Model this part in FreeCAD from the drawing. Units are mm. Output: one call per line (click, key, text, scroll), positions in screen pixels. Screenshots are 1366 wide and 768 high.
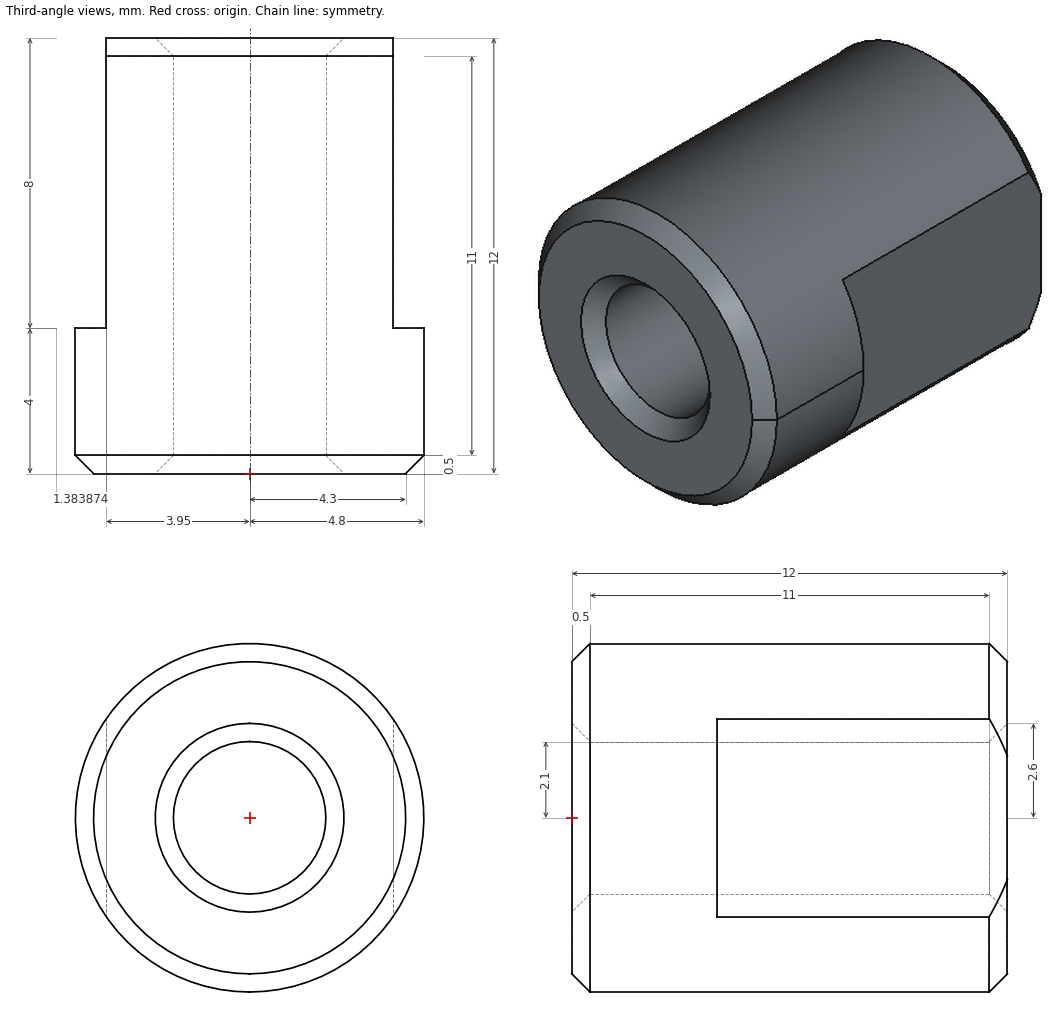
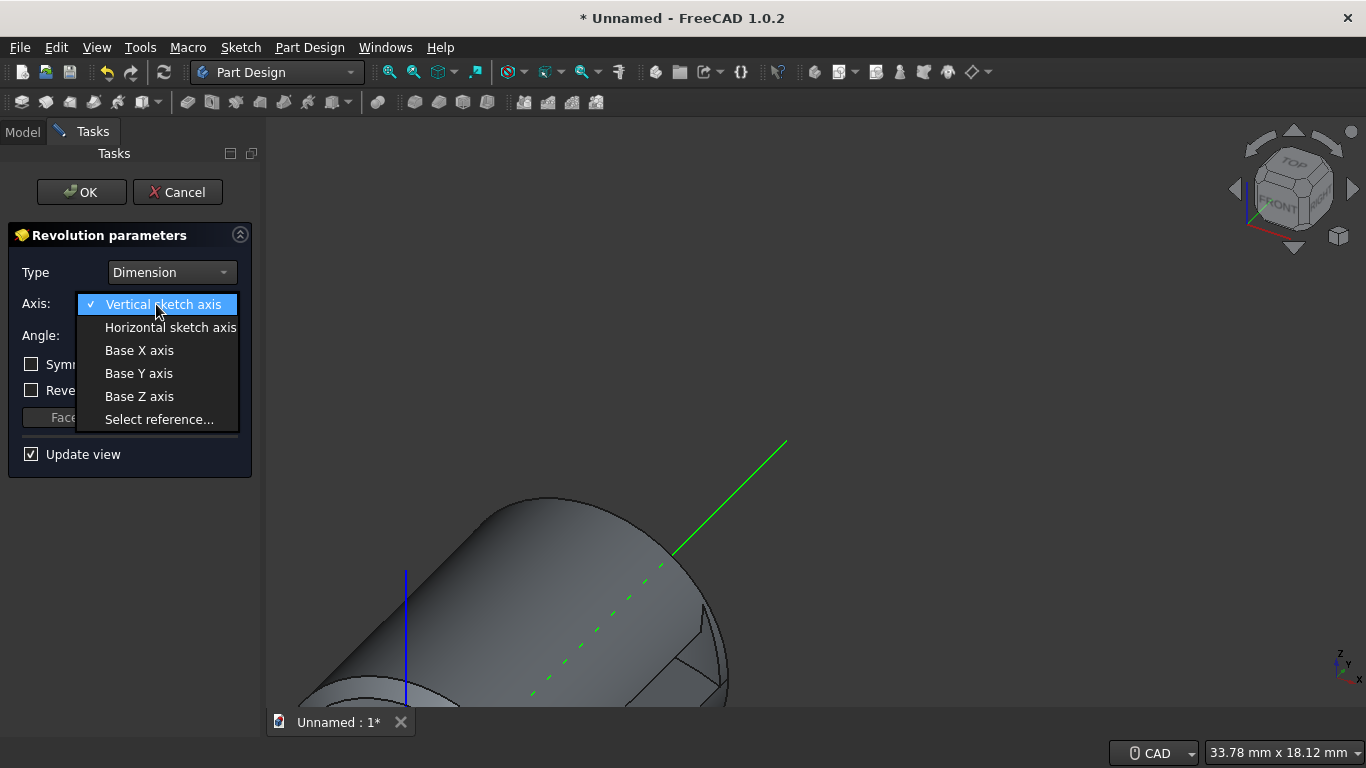
click(156, 328)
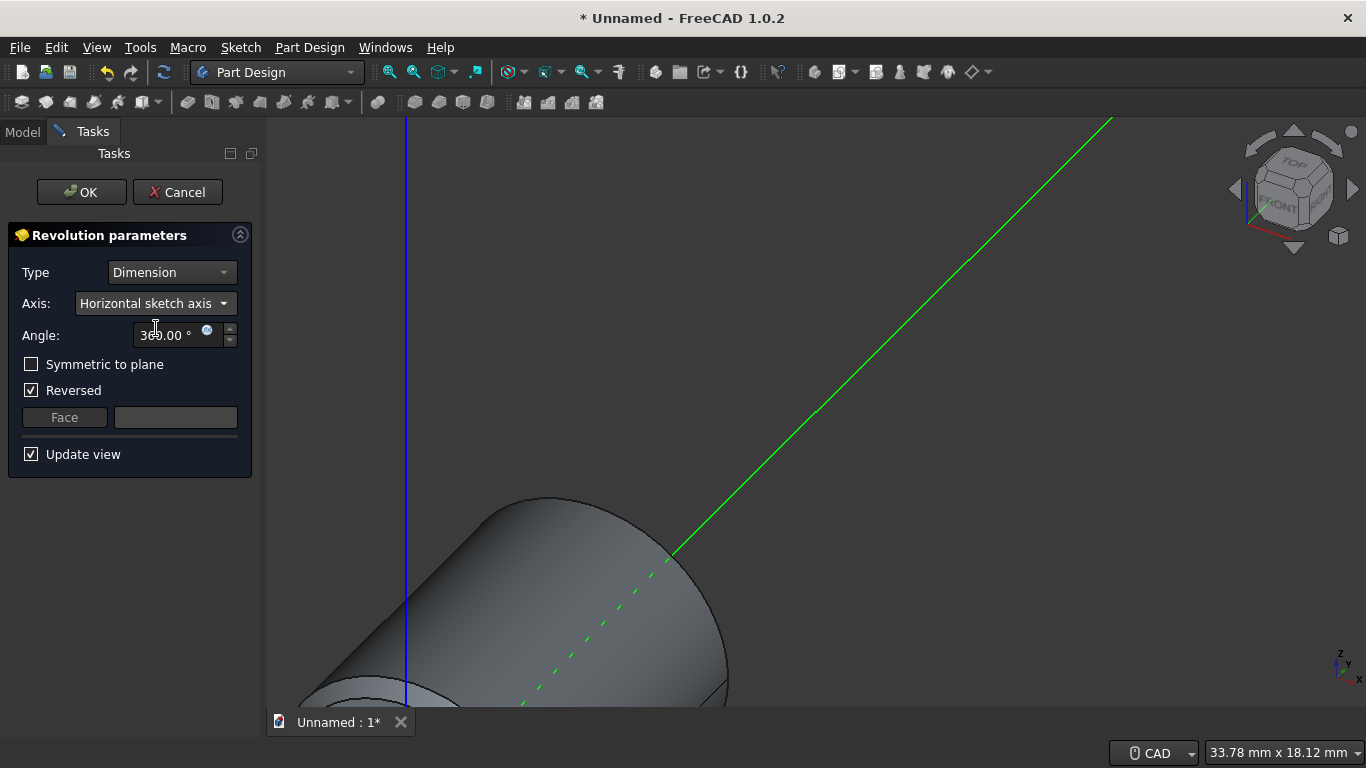
click(82, 192)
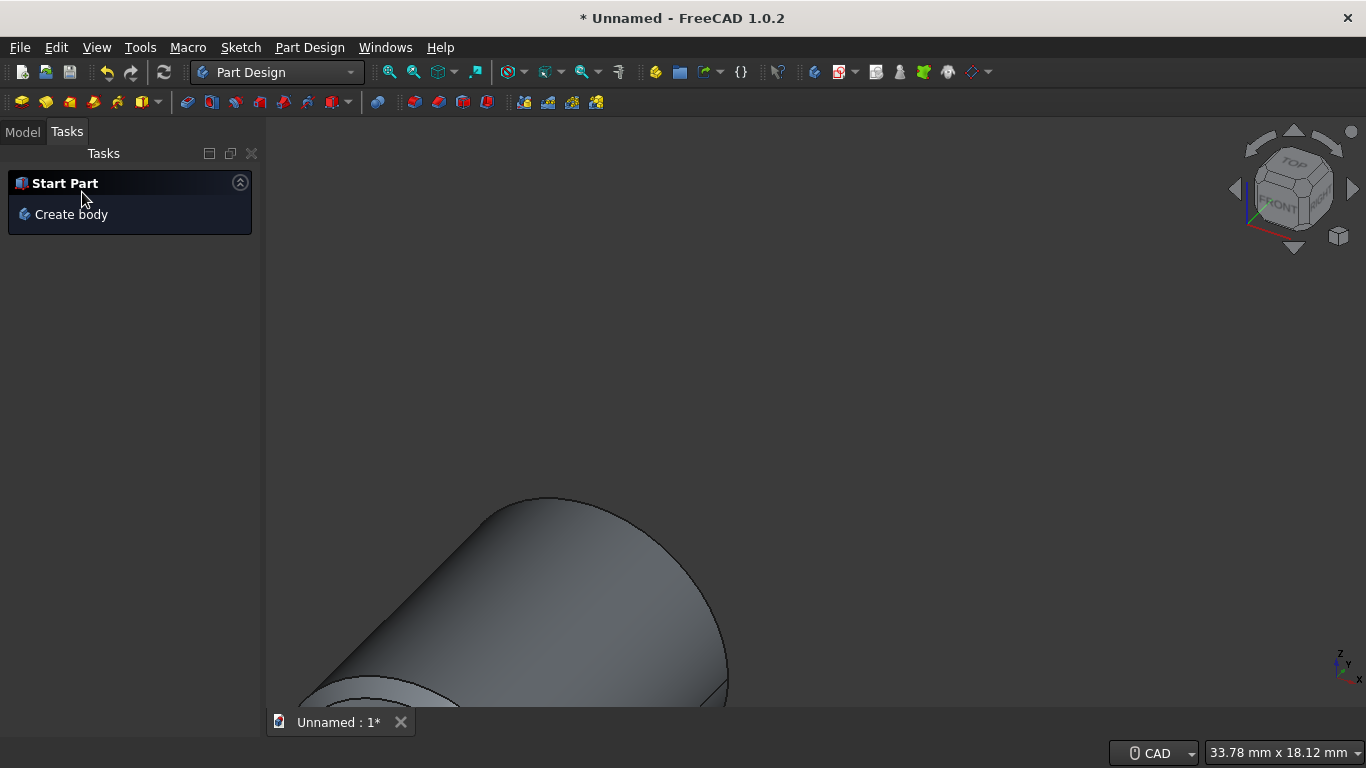
click(390, 72)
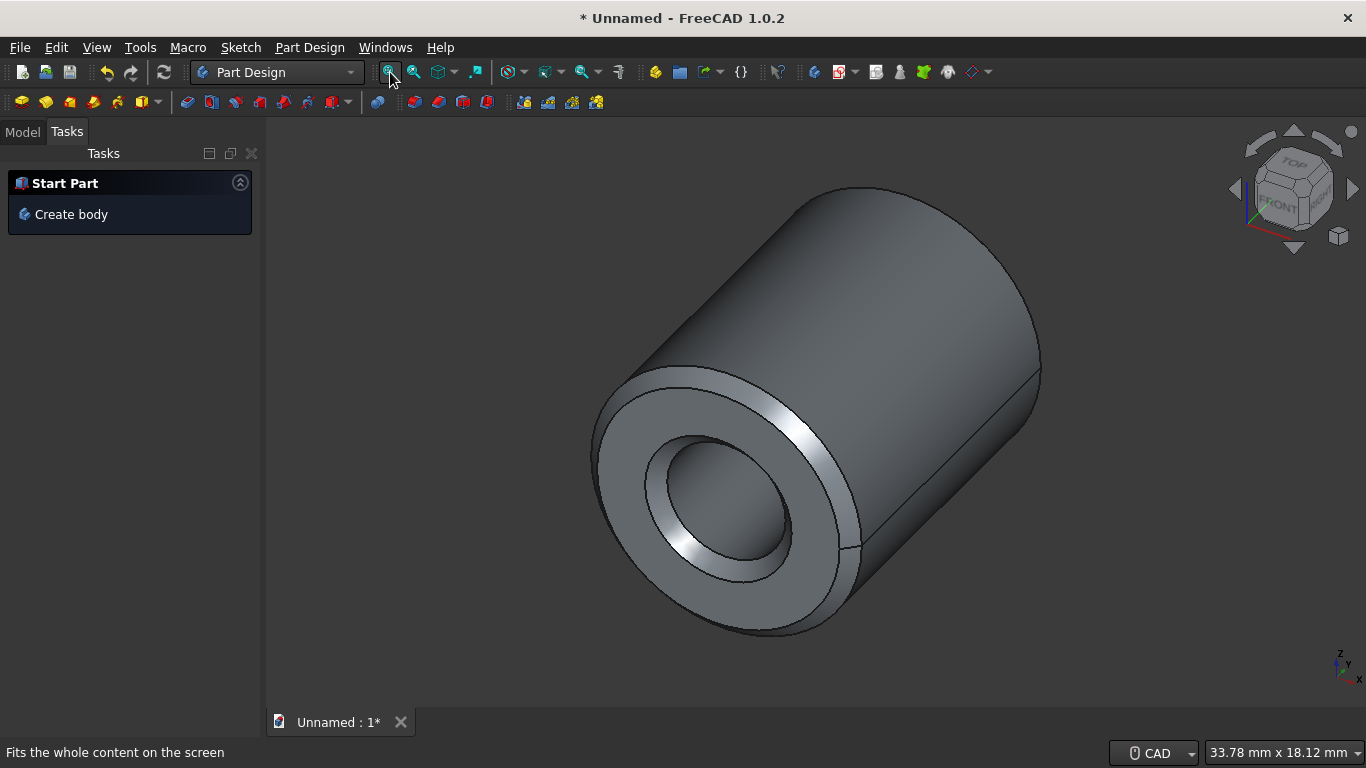
click(840, 72)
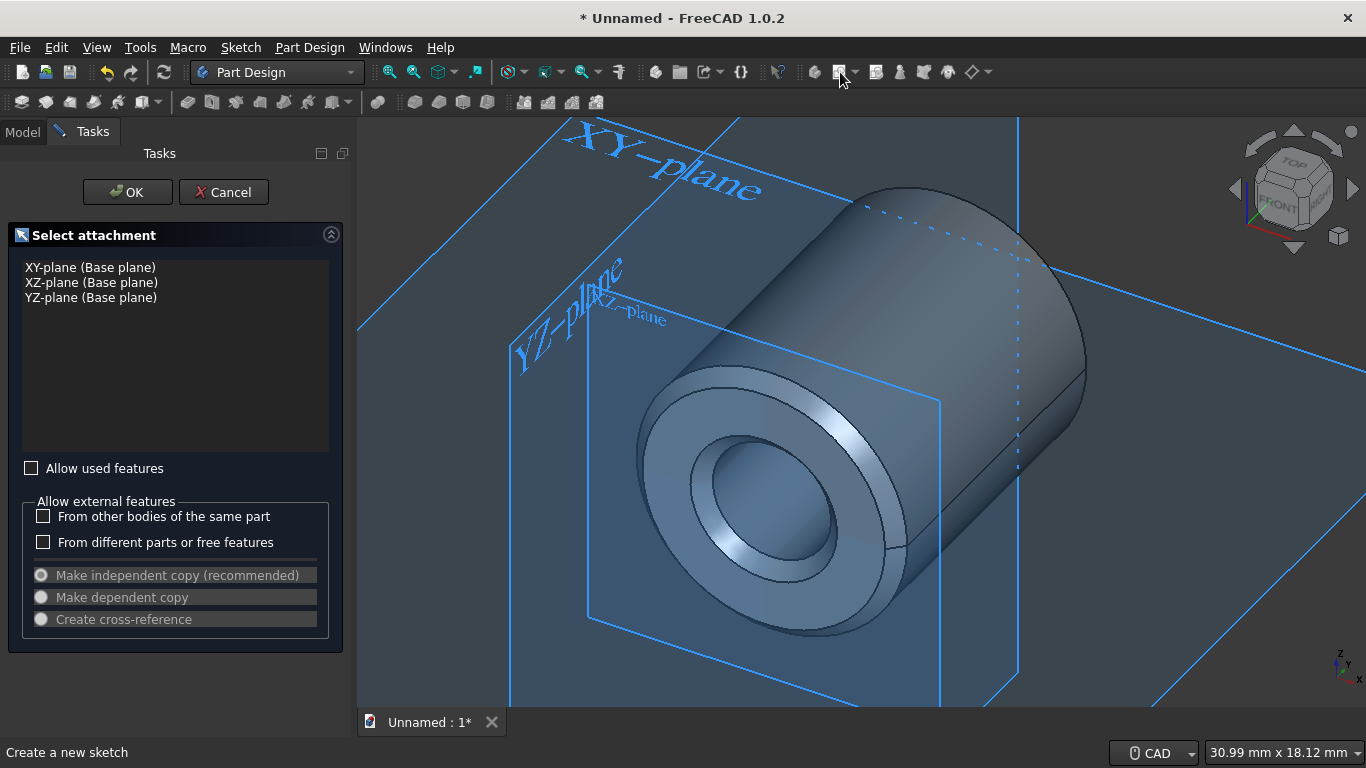
click(82, 268)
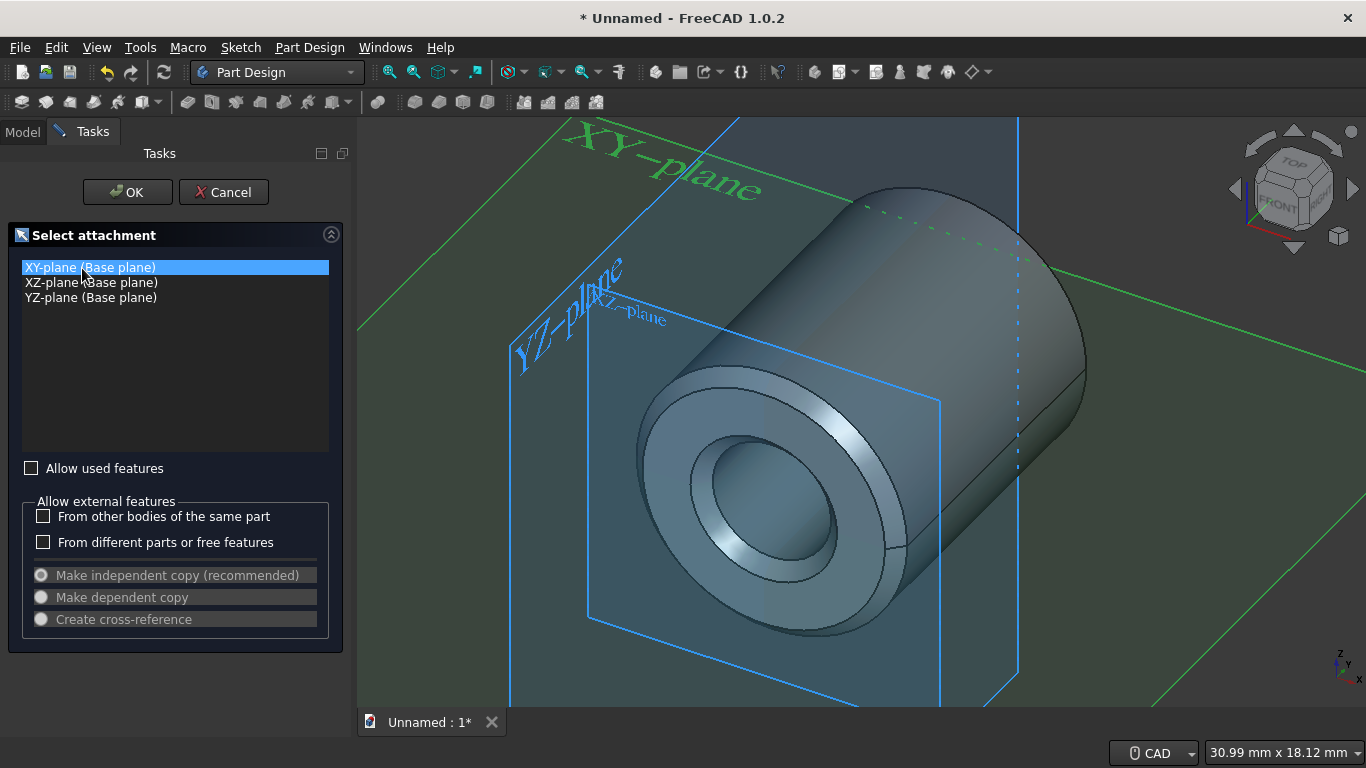
click(128, 192)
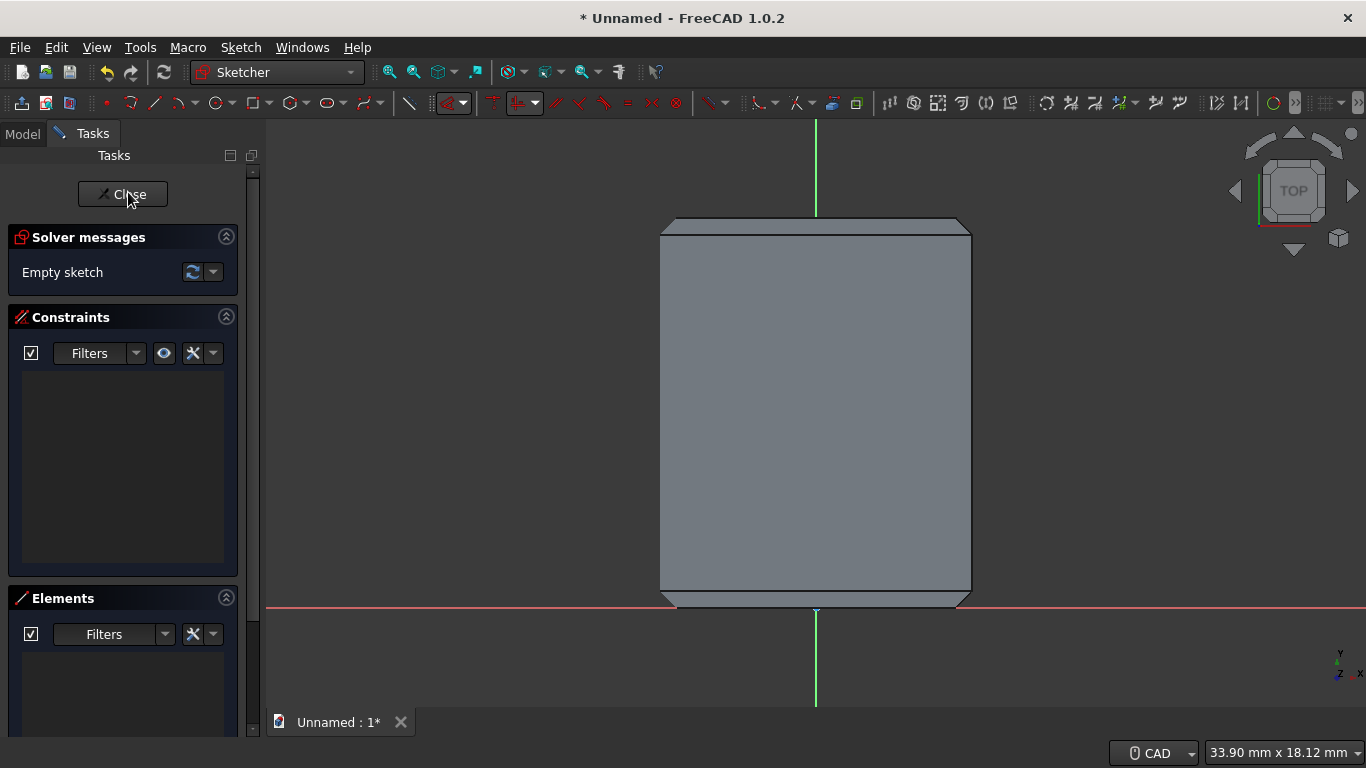
click(70, 104)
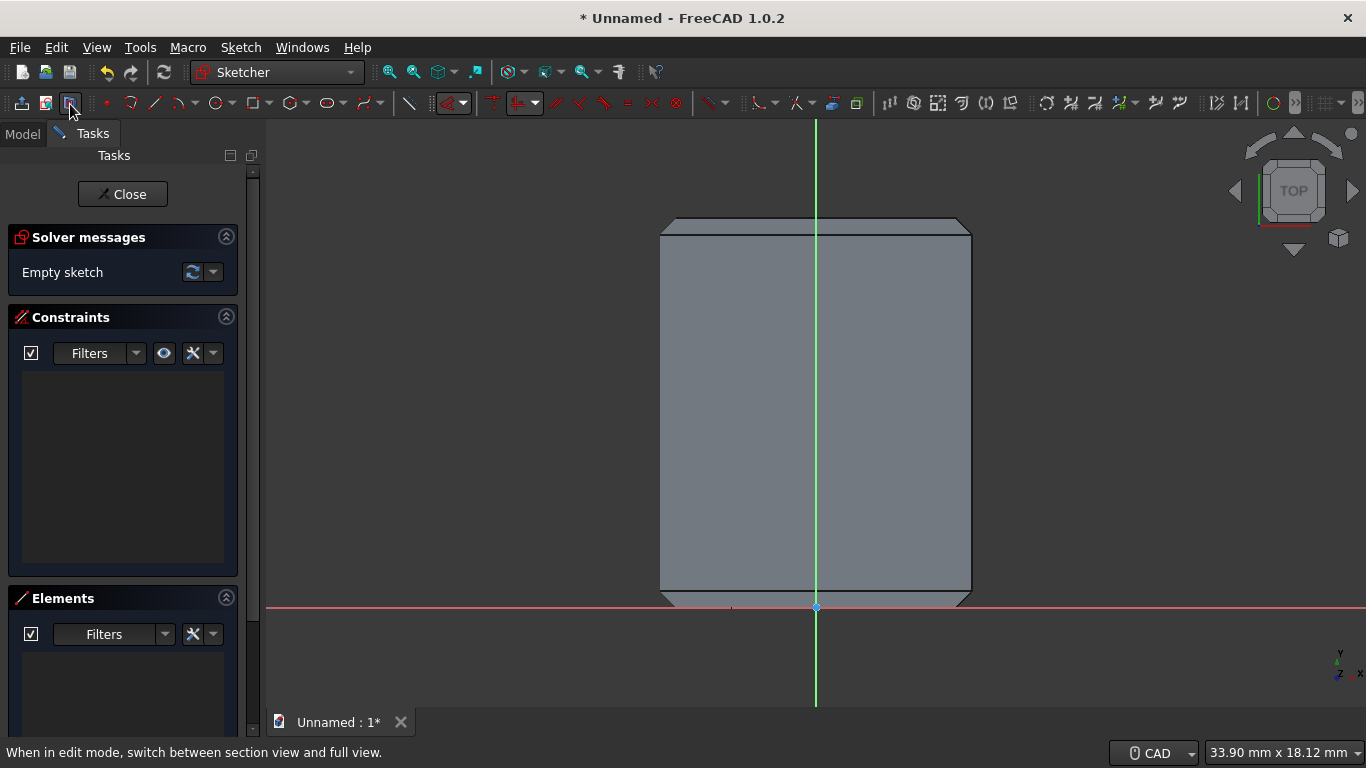
click(254, 104)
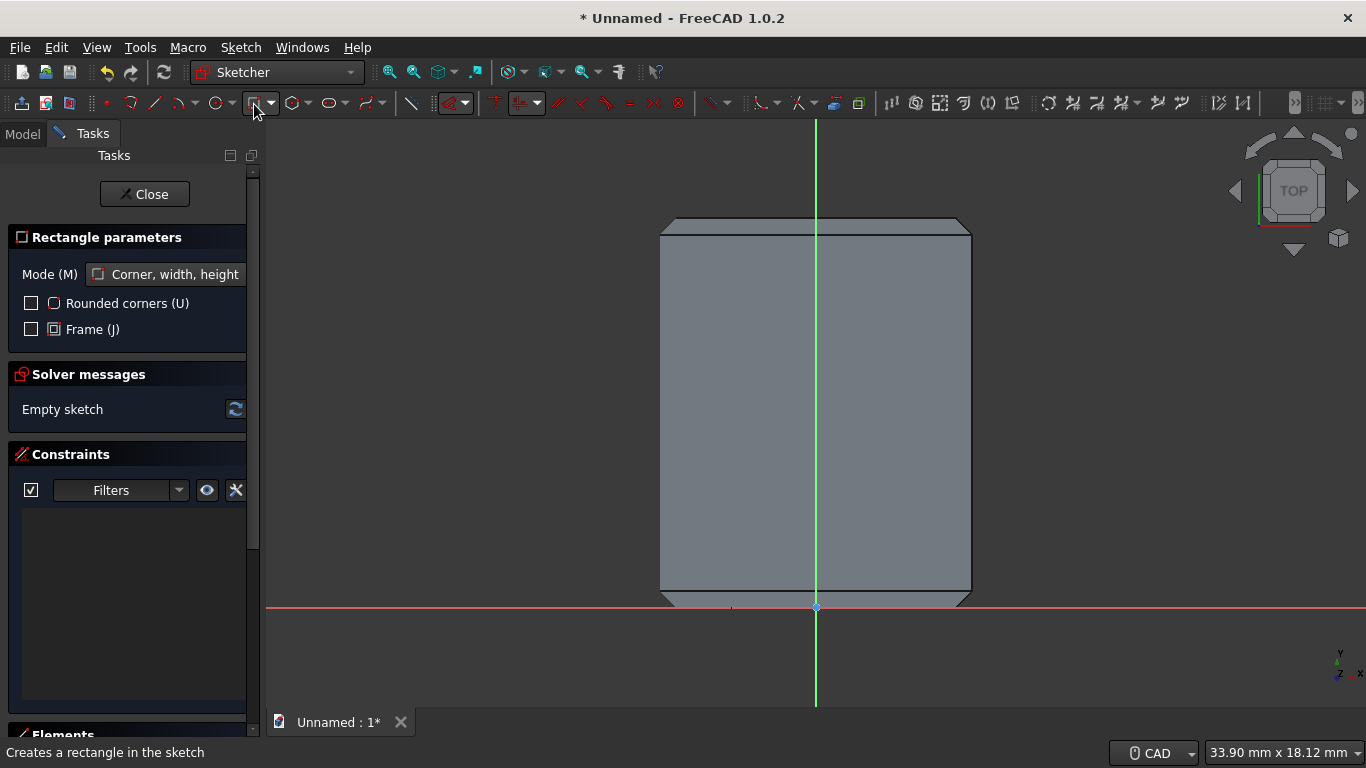
click(643, 218)
click(688, 478)